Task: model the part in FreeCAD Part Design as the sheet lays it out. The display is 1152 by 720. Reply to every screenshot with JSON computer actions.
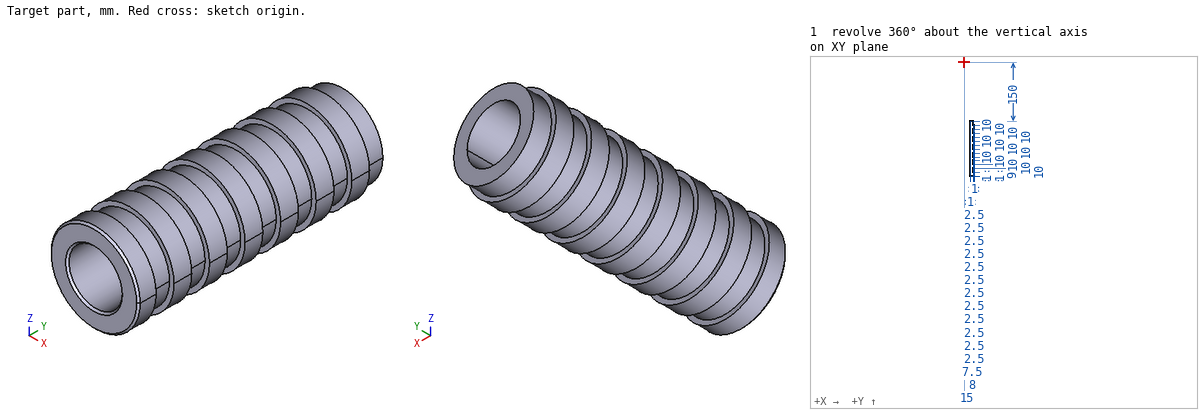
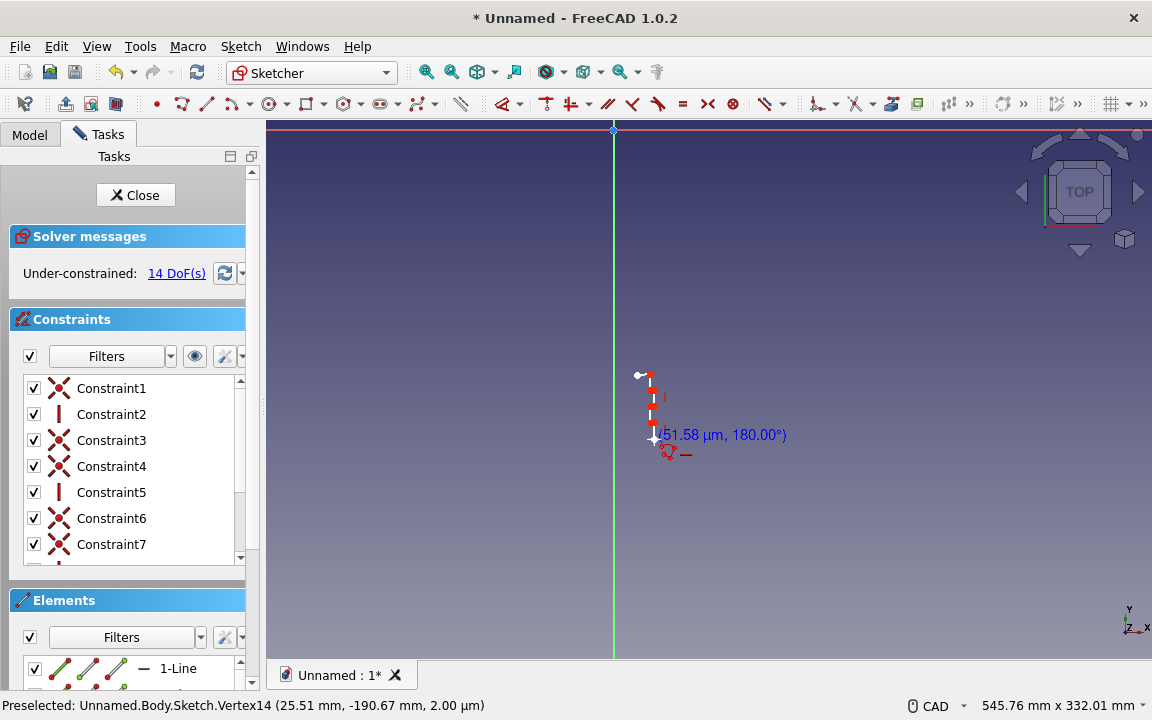
{"action": "scroll", "coordinate": [650, 439], "scroll_direction": "up", "scroll_amount": 7}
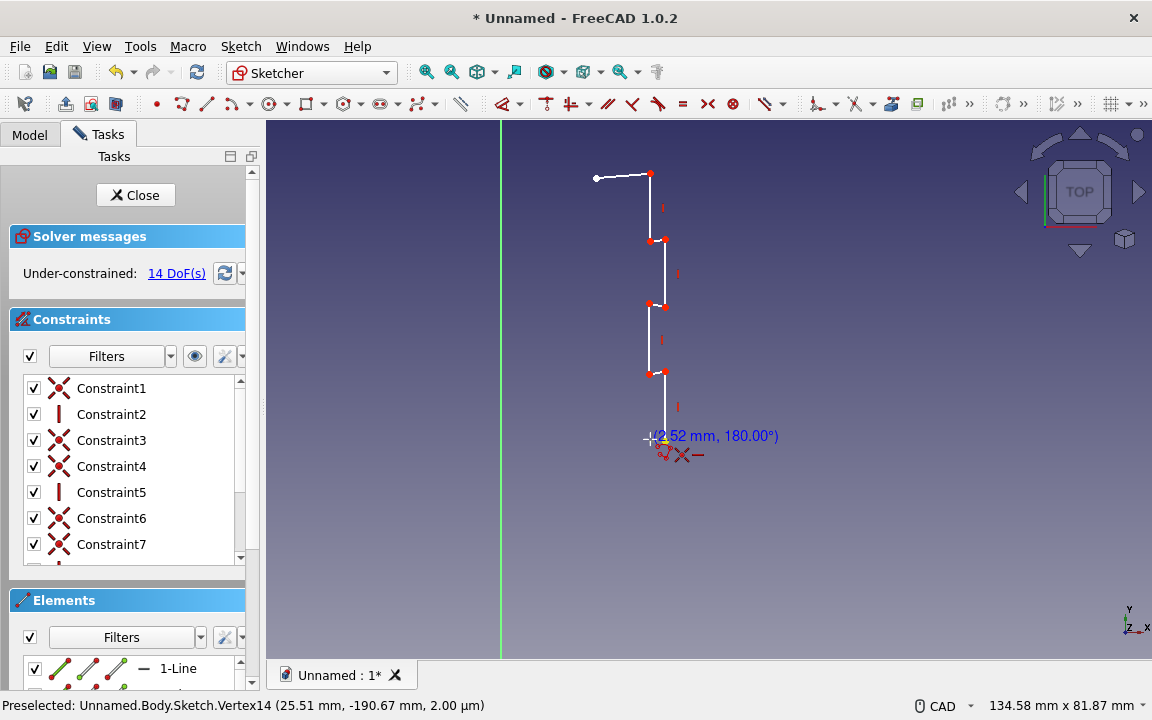
{"action": "left_click", "coordinate": [649, 437]}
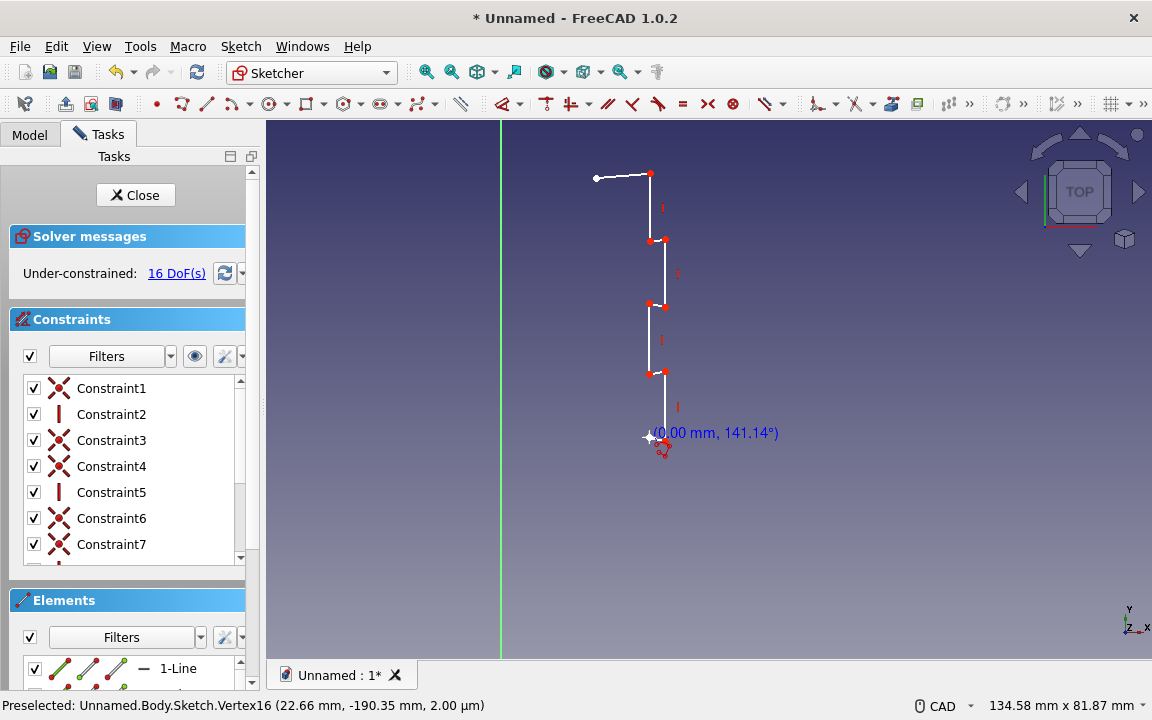
{"action": "scroll", "coordinate": [652, 439], "scroll_direction": "down", "scroll_amount": 9}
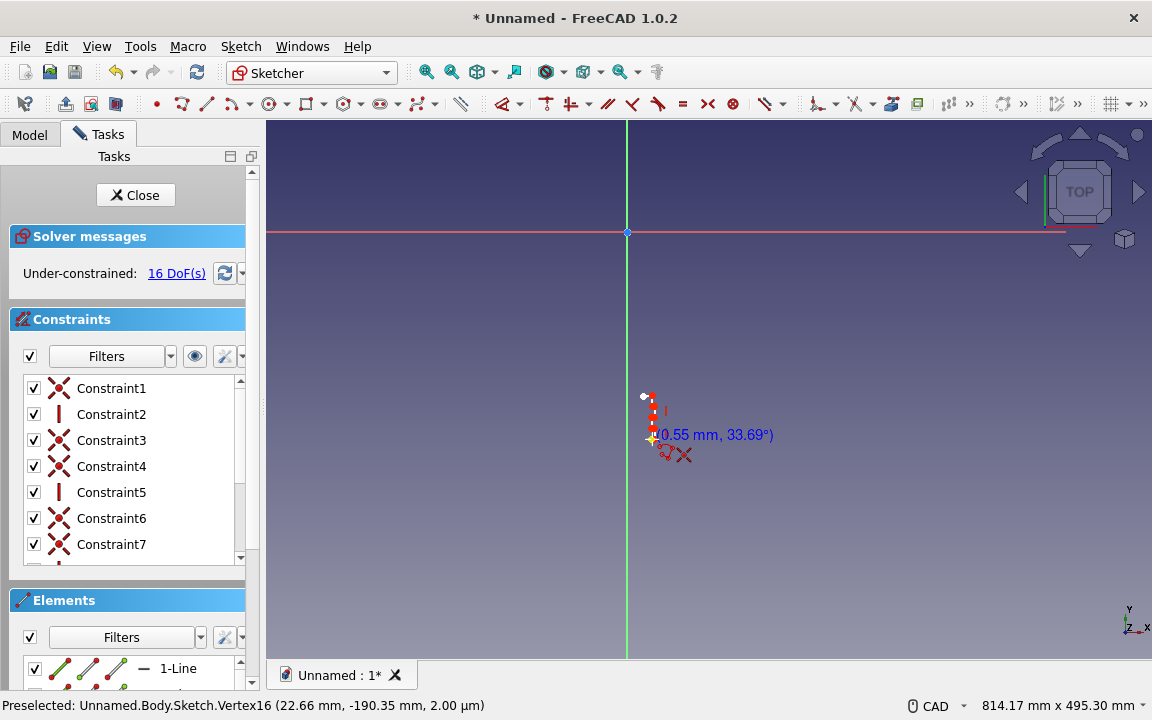
{"action": "scroll", "coordinate": [652, 450], "scroll_direction": "up", "scroll_amount": 2}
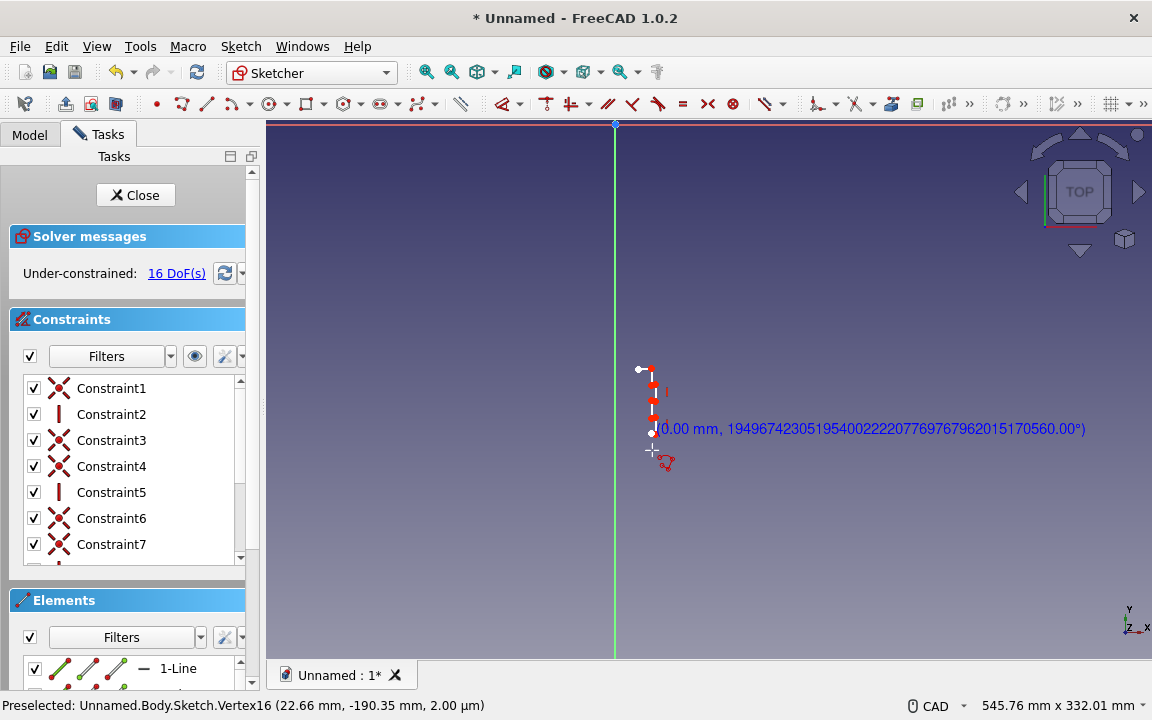
{"action": "left_click", "coordinate": [652, 450]}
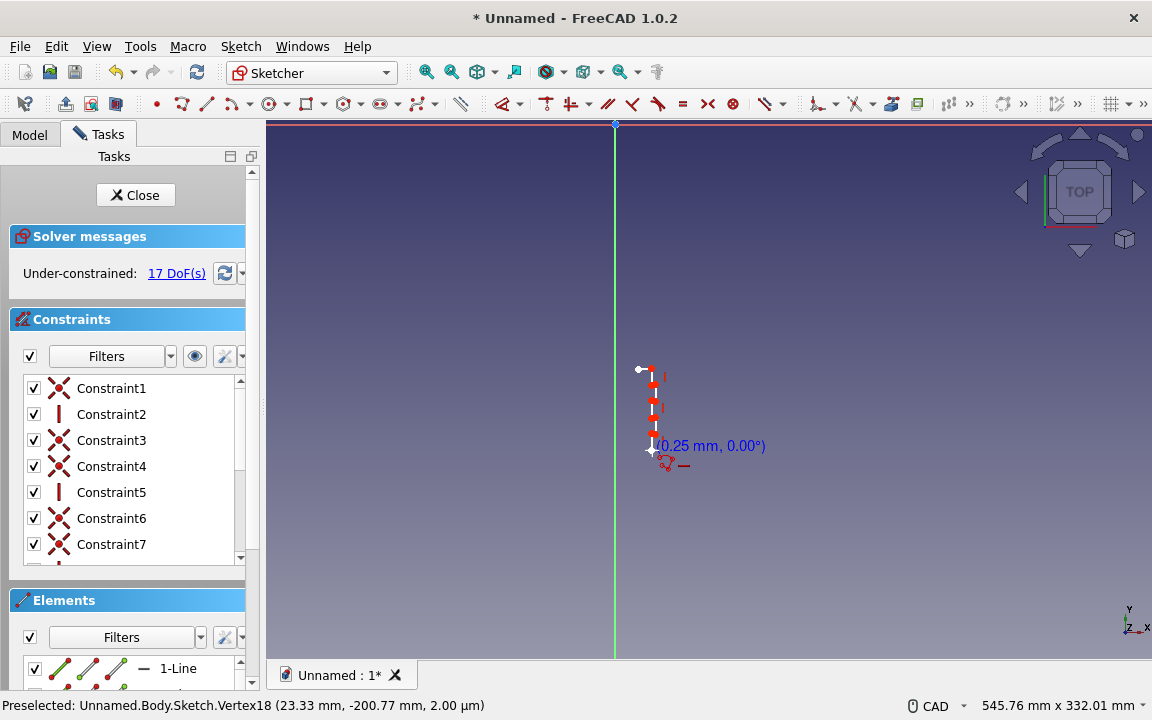
{"action": "scroll", "coordinate": [656, 450], "scroll_direction": "up", "scroll_amount": 7}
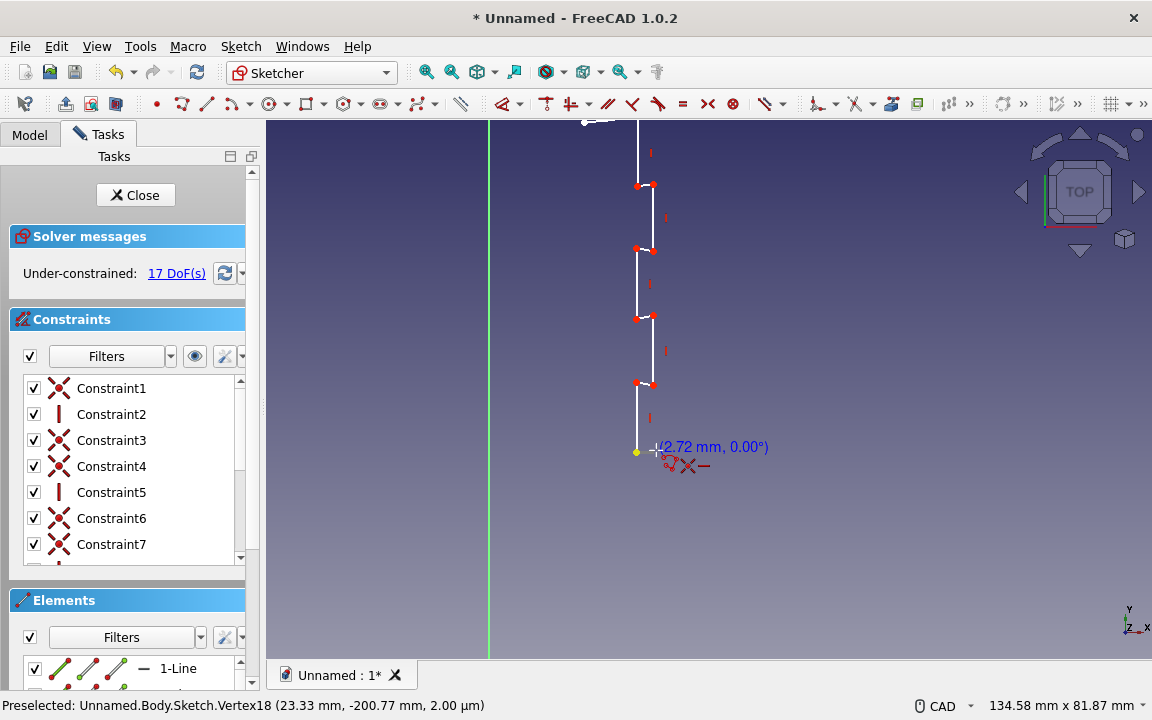
{"action": "left_click", "coordinate": [653, 448]}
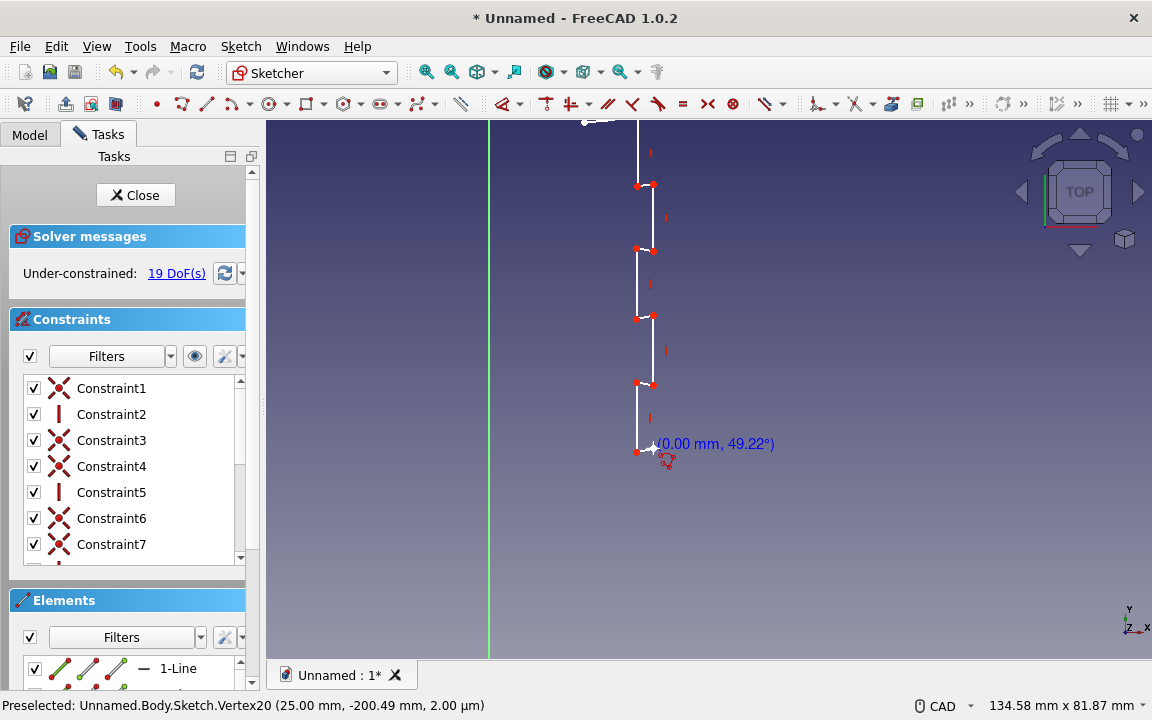
{"action": "scroll", "coordinate": [654, 450], "scroll_direction": "down", "scroll_amount": 9}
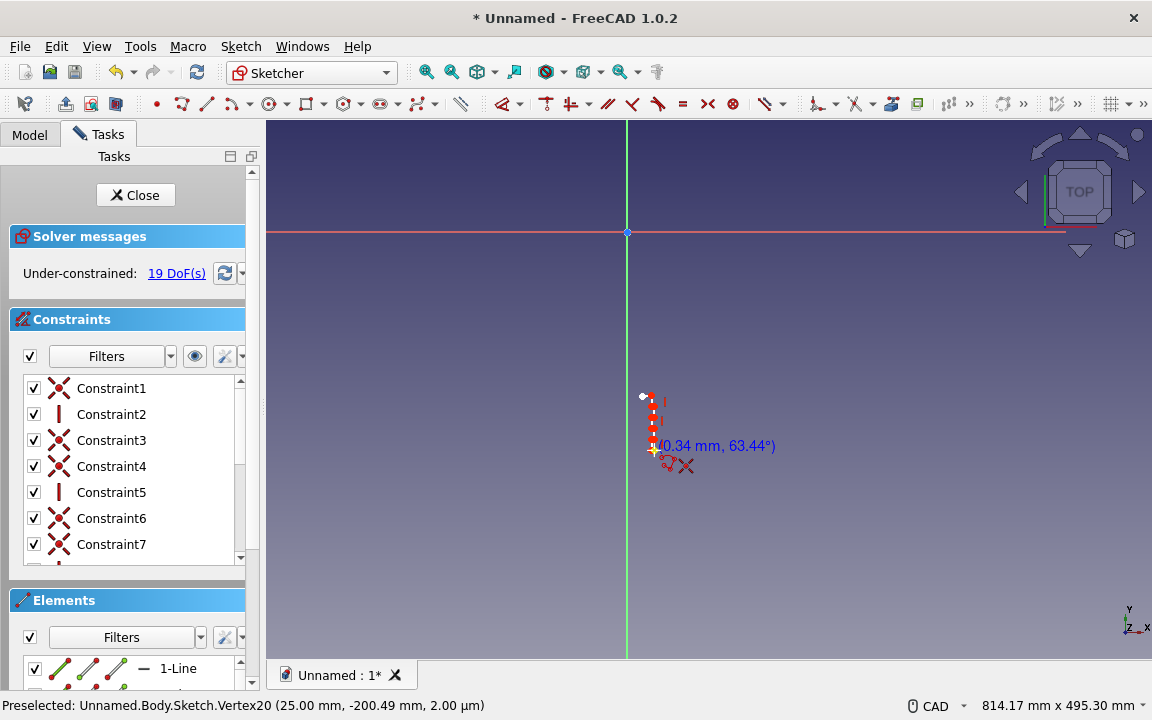
{"action": "scroll", "coordinate": [654, 461], "scroll_direction": "up", "scroll_amount": 2}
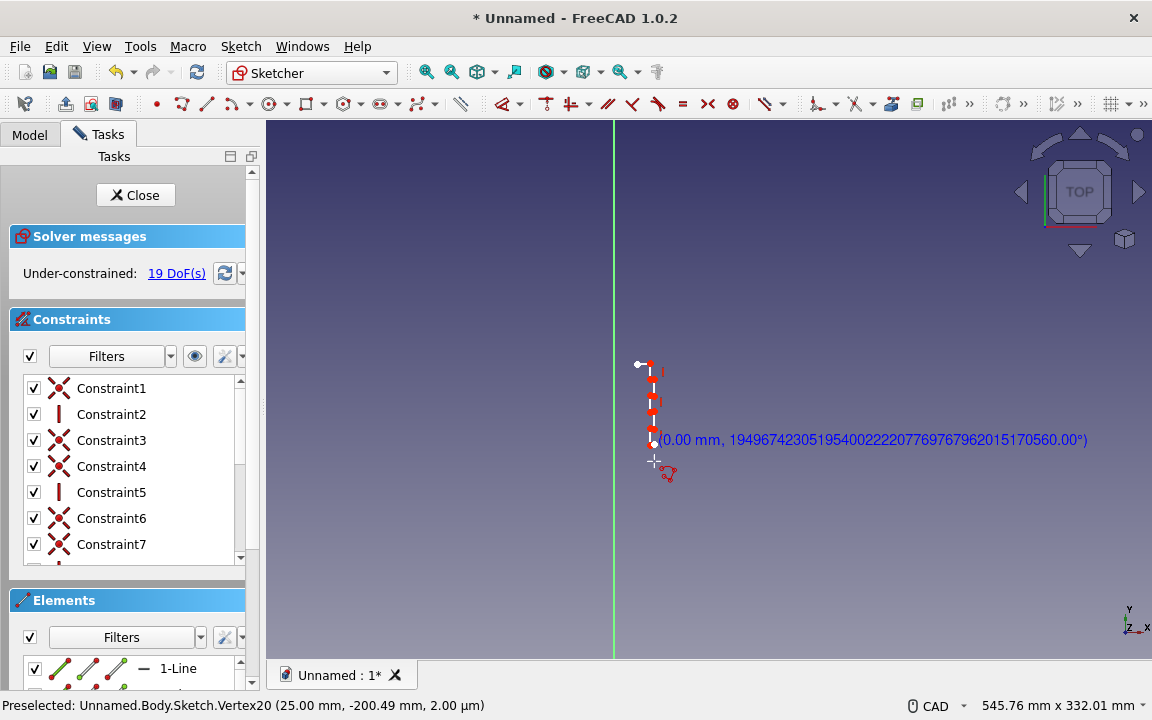
{"action": "left_click", "coordinate": [654, 461]}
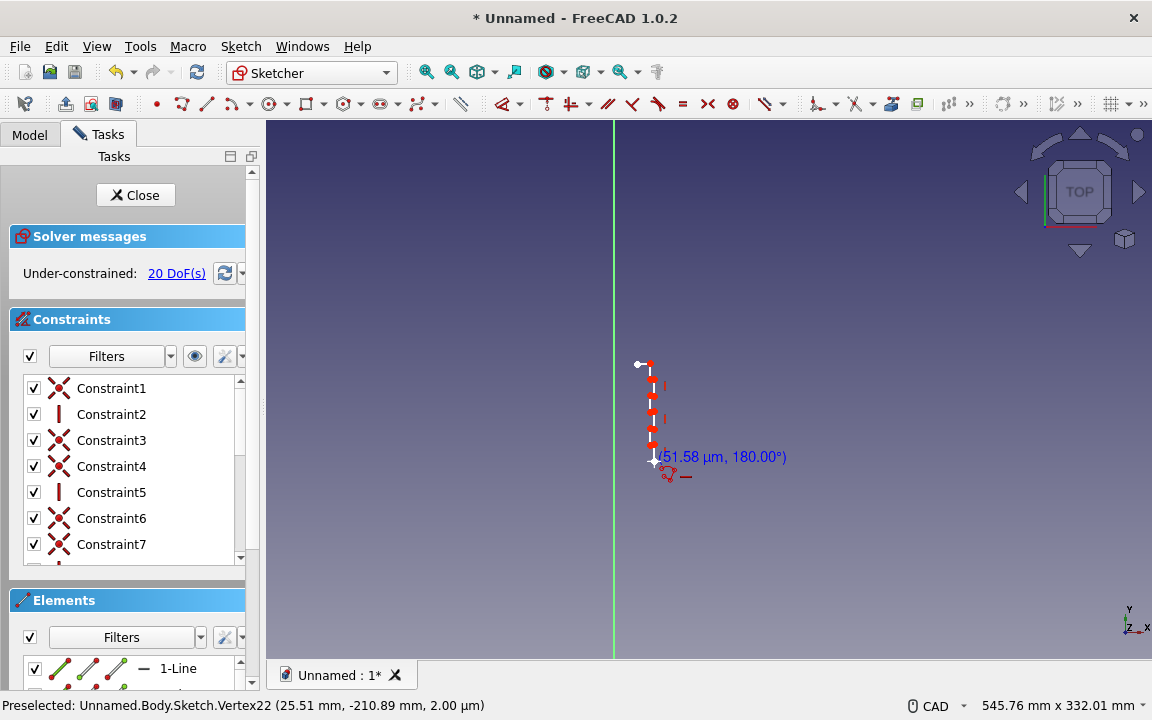
{"action": "scroll", "coordinate": [650, 461], "scroll_direction": "up", "scroll_amount": 7}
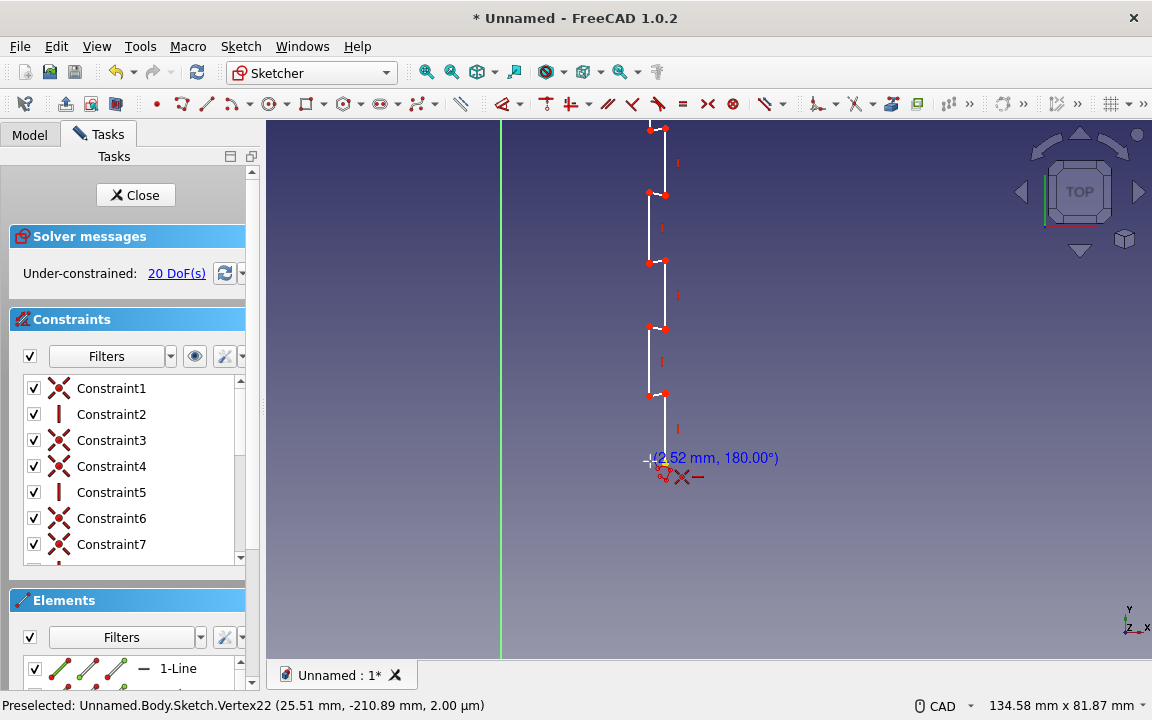
{"action": "left_click", "coordinate": [649, 459]}